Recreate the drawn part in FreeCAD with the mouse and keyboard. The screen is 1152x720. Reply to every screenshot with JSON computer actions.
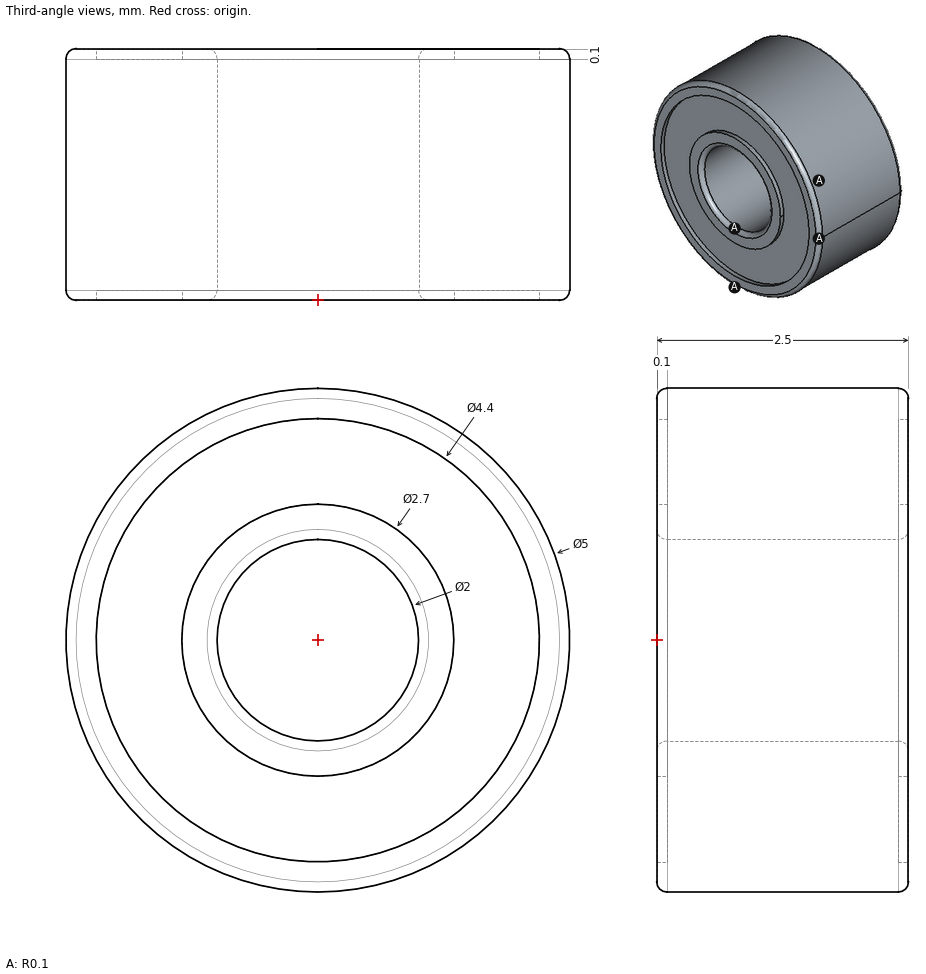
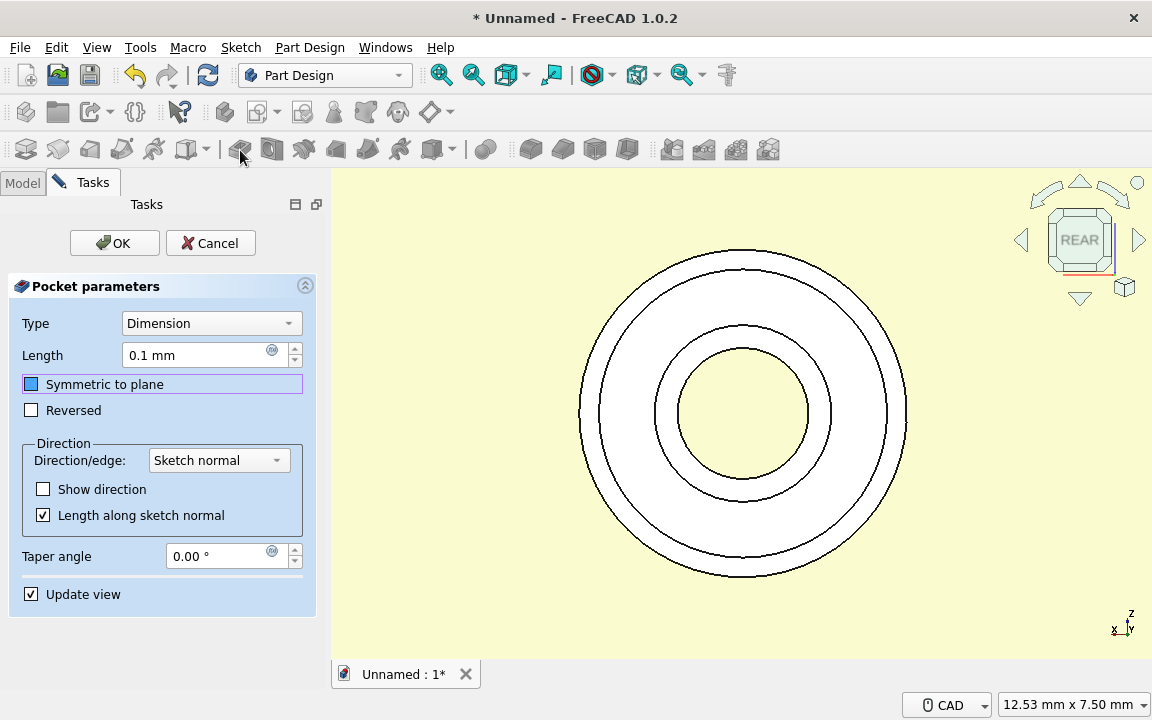
{"action": "left_click", "coordinate": [30, 410]}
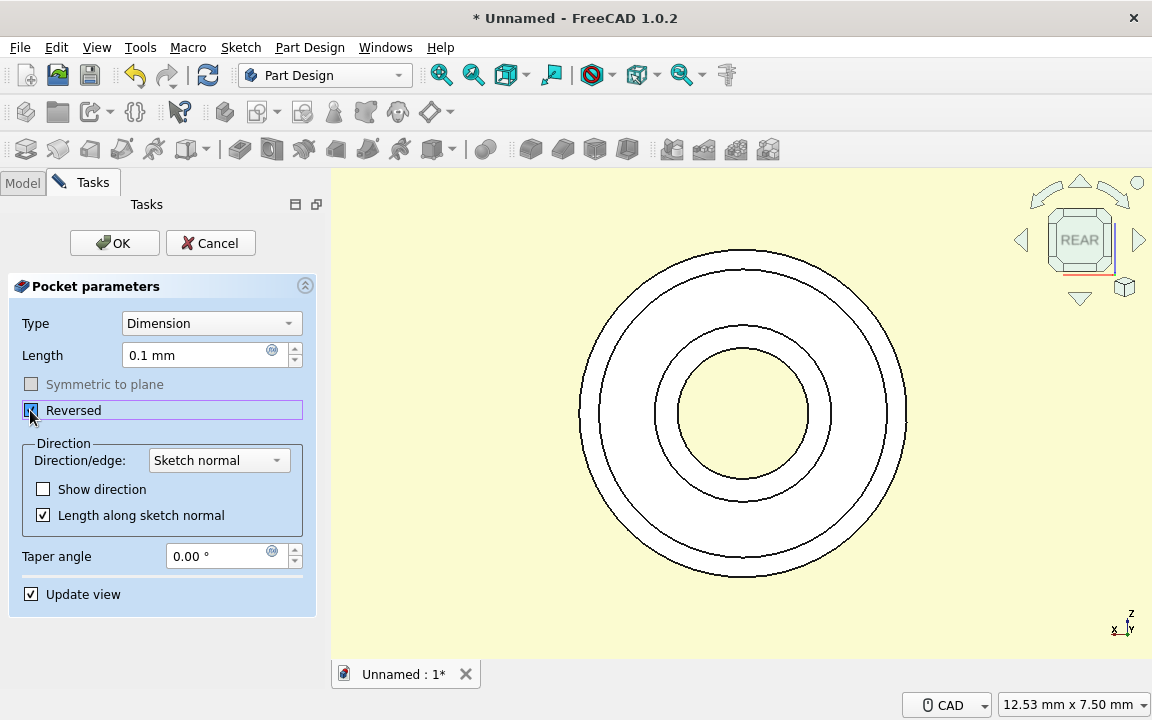
{"action": "left_click", "coordinate": [115, 243]}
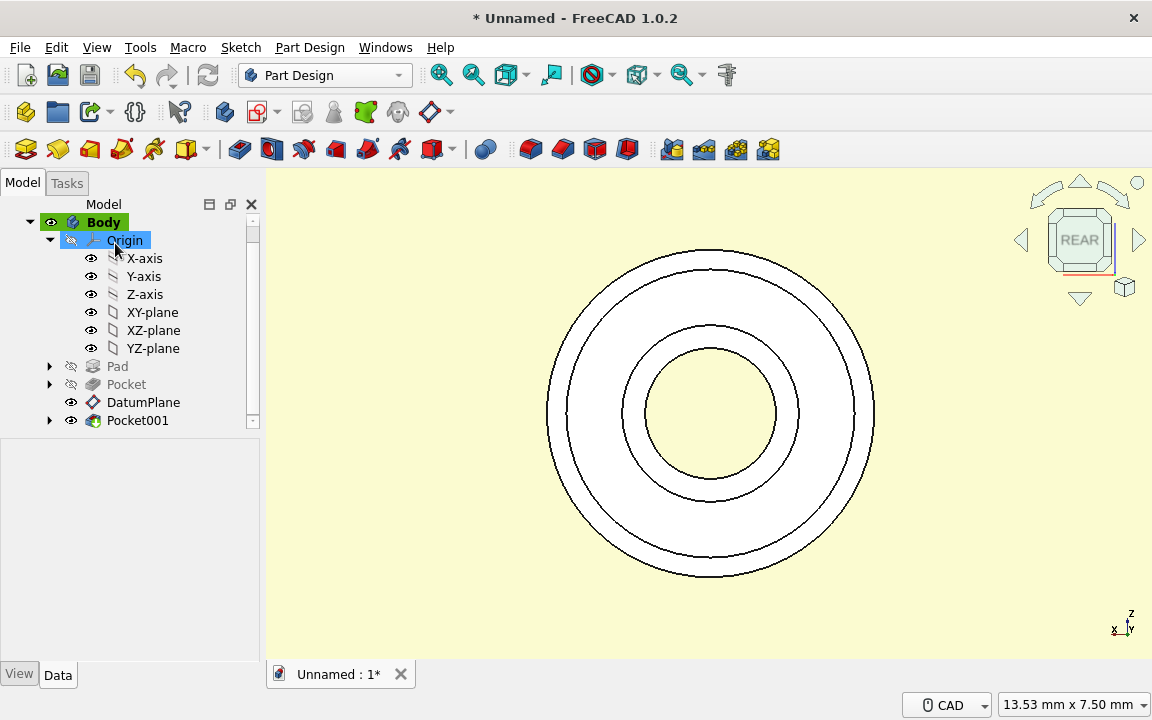
{"action": "left_click", "coordinate": [116, 402]}
{"action": "key", "text": "space"}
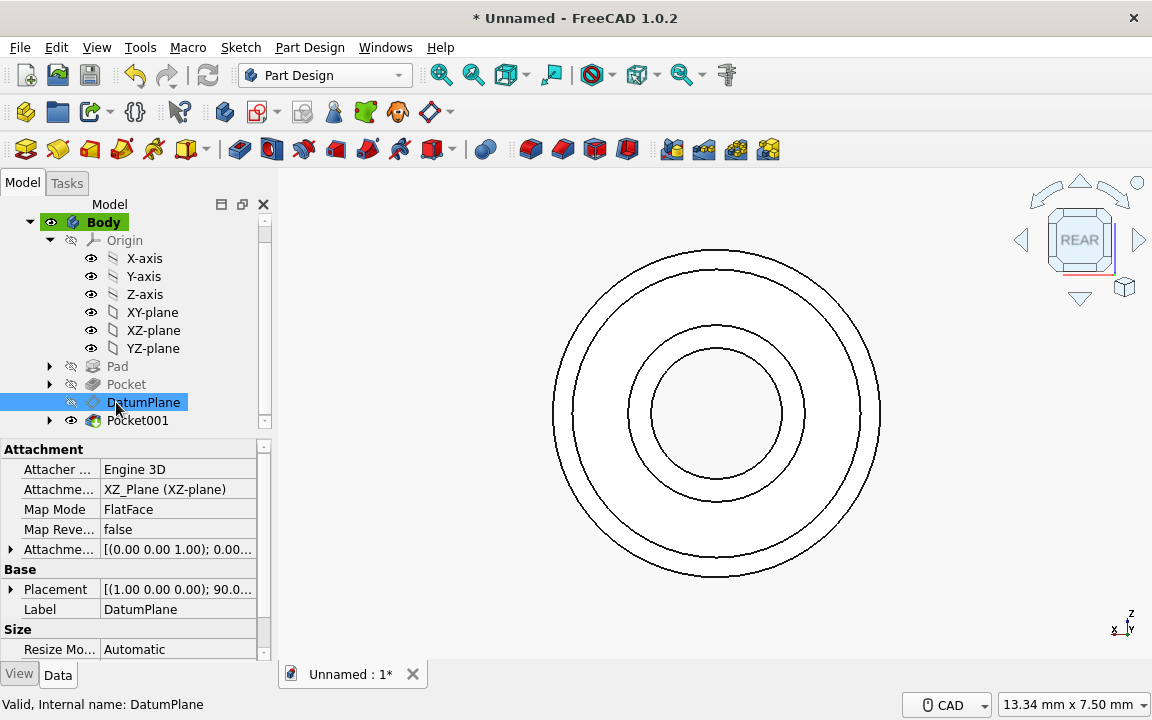
{"action": "left_click", "coordinate": [880, 413]}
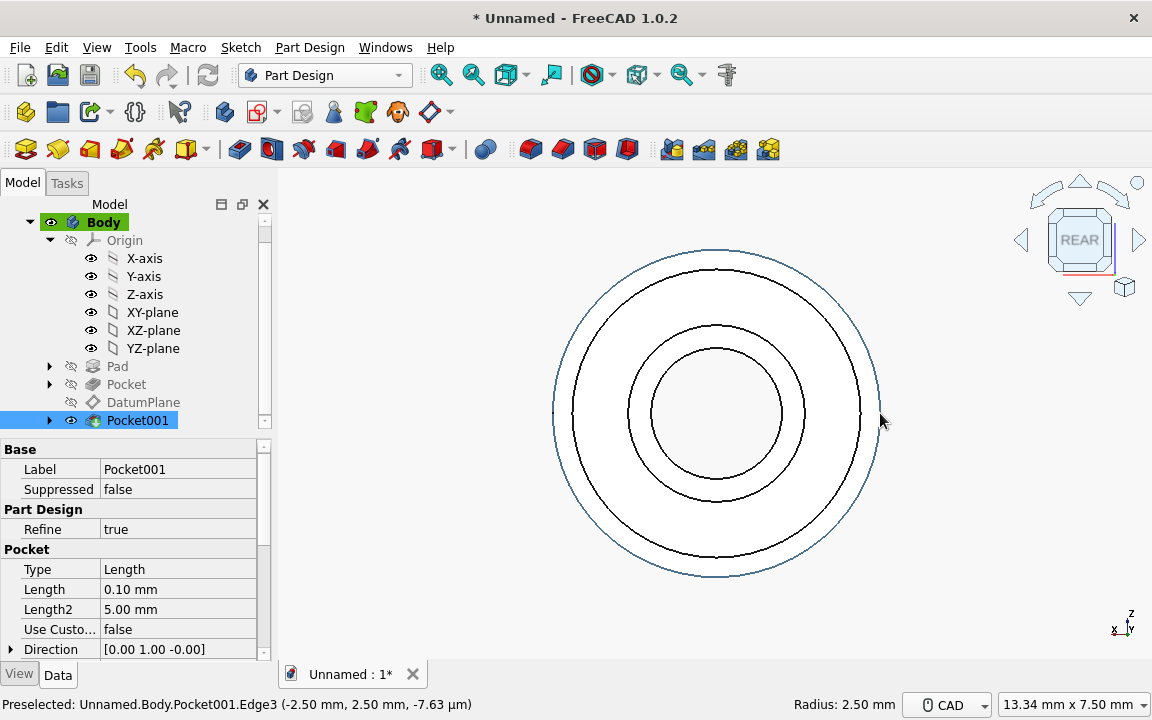
{"action": "left_click", "coordinate": [770, 374], "text": "ctrl"}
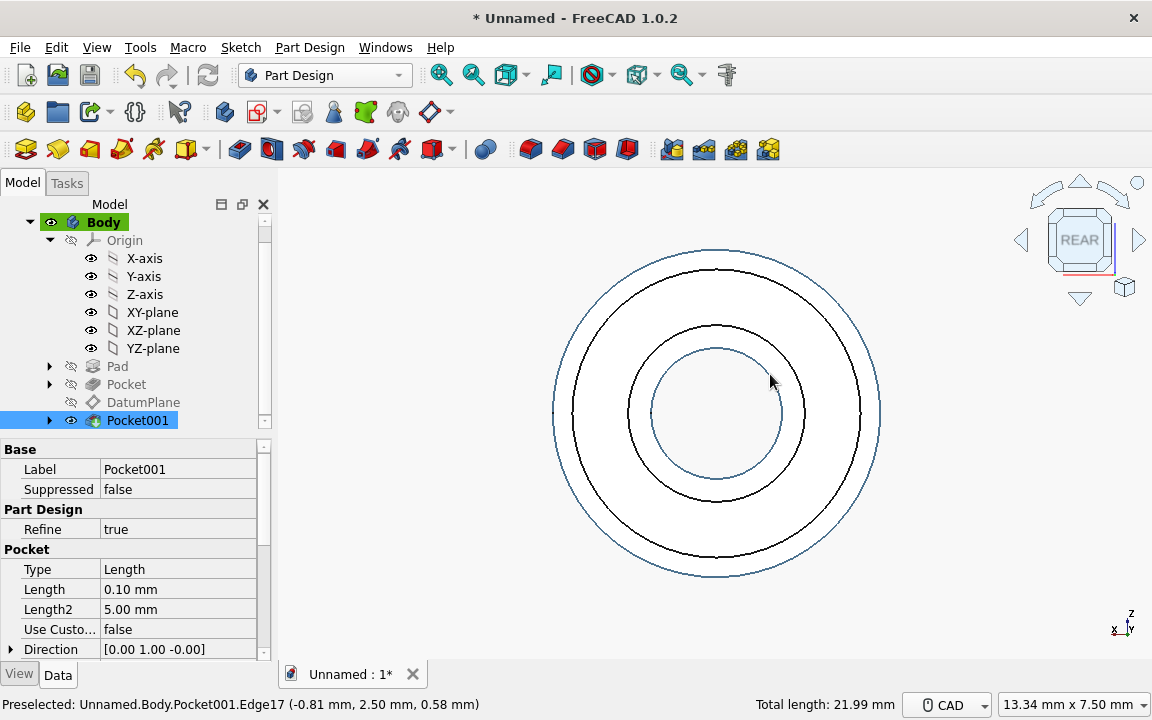
{"action": "key", "text": "0"}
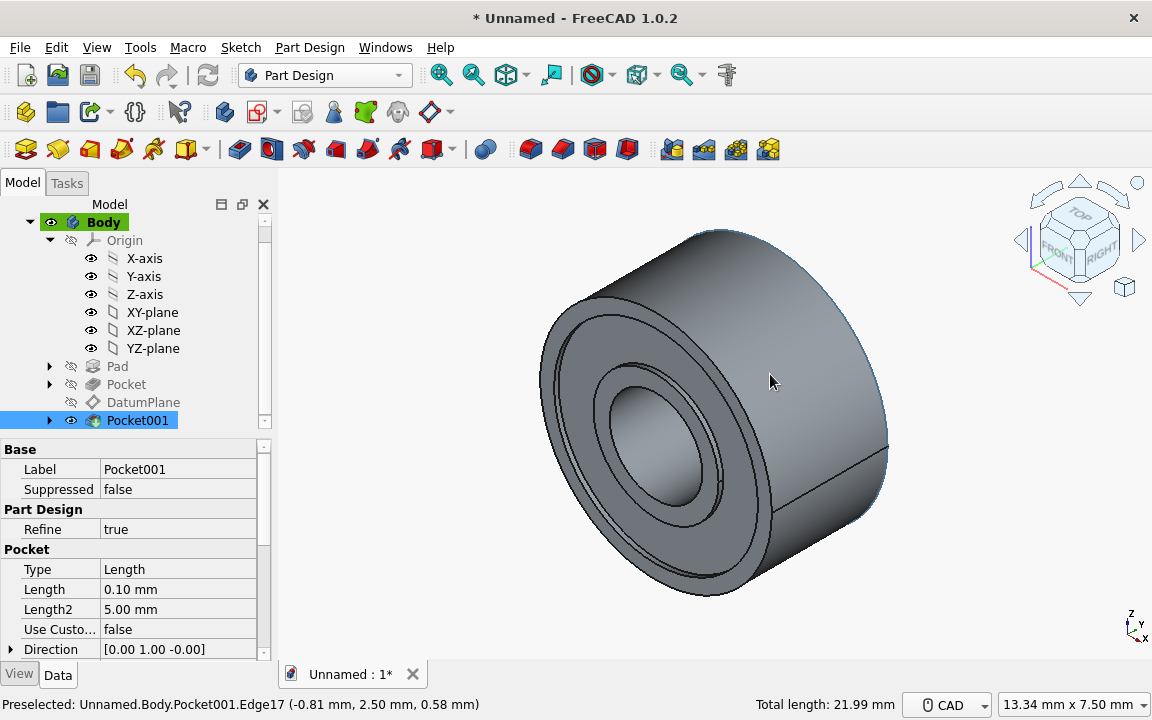
{"action": "left_click", "coordinate": [562, 313], "text": "ctrl"}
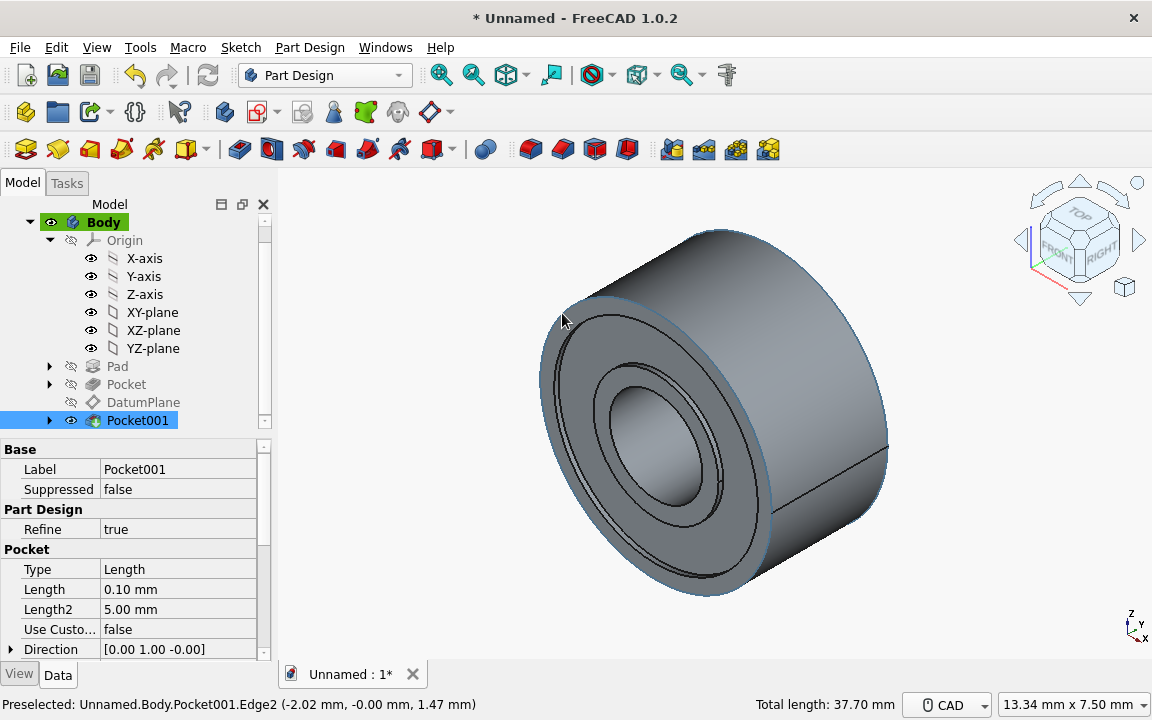
{"action": "left_click", "coordinate": [610, 419], "text": "ctrl"}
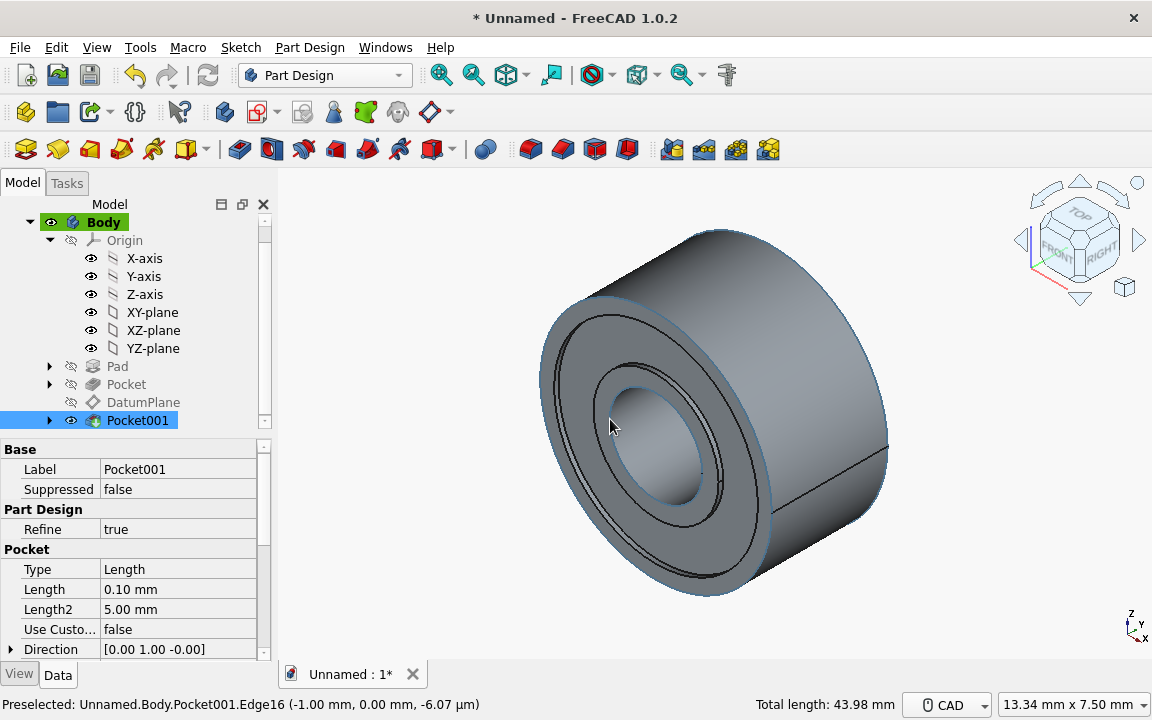
{"action": "left_click", "coordinate": [532, 150]}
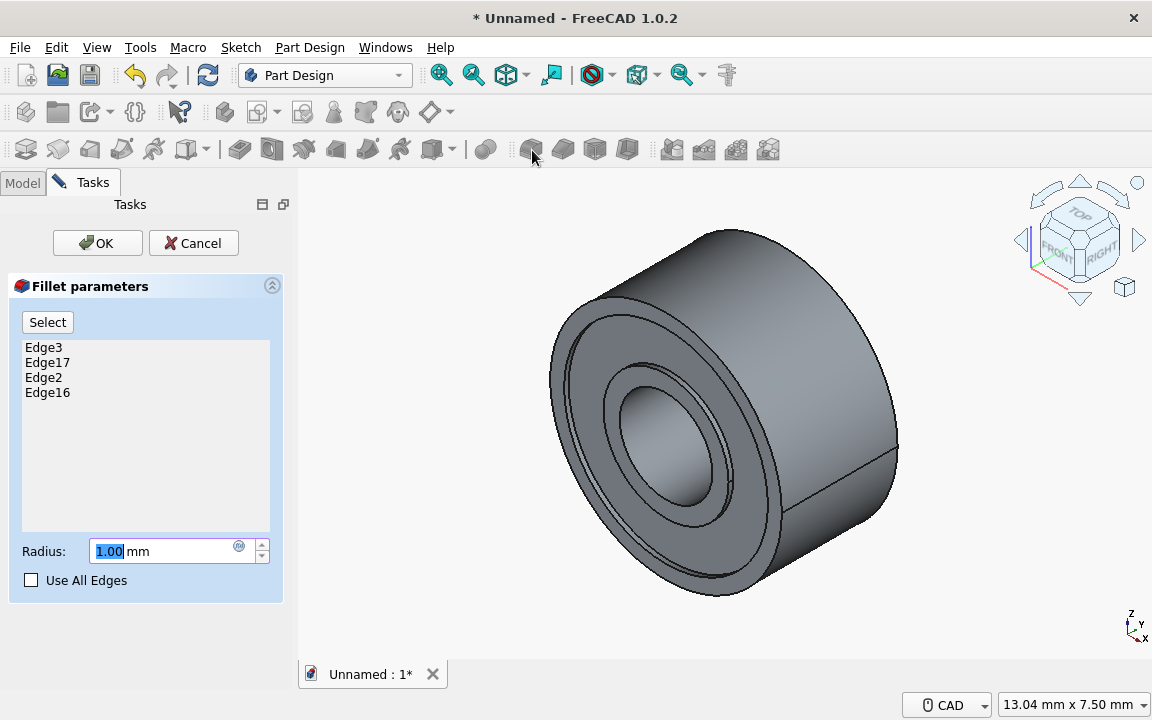
{"action": "type", "text": "0.1"}
{"action": "key", "text": "Tab"}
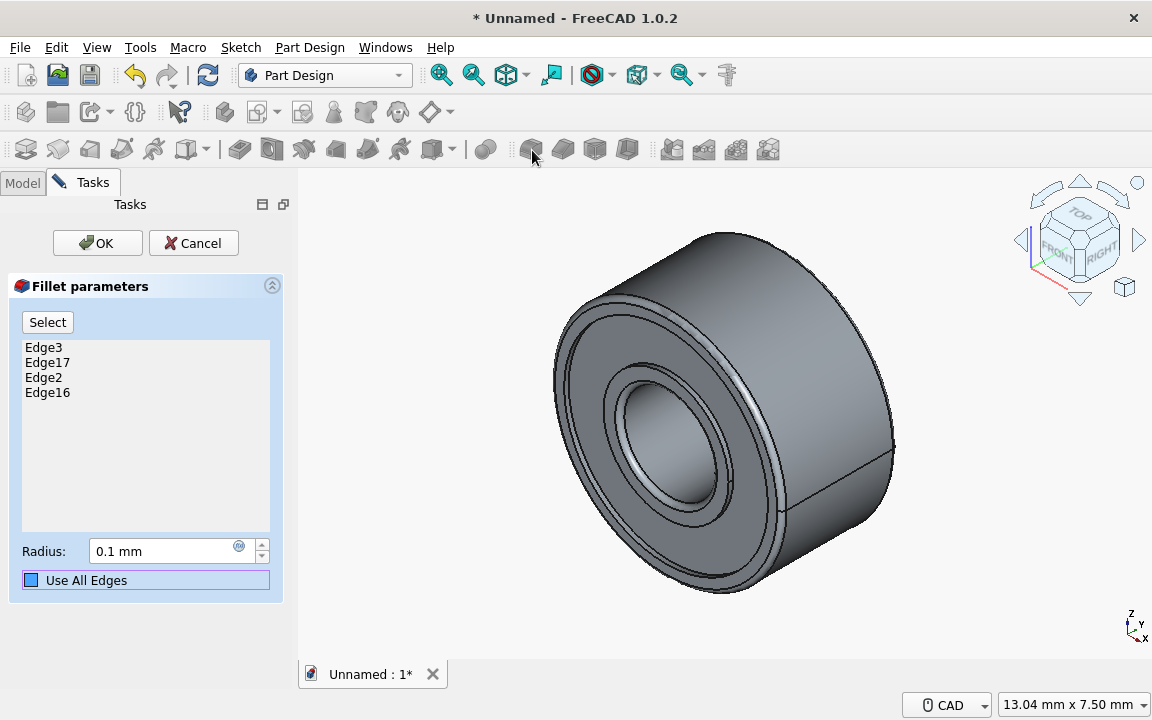
{"action": "left_click", "coordinate": [98, 243]}